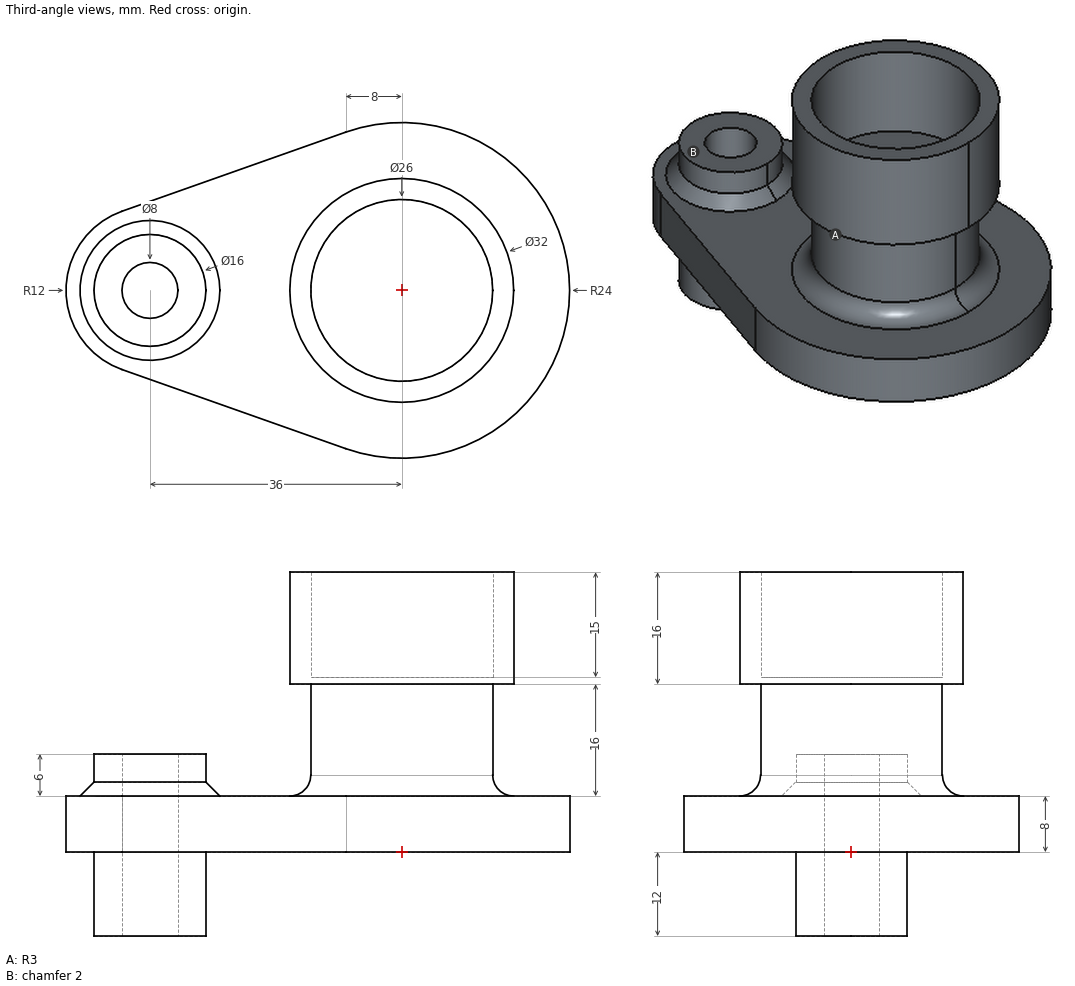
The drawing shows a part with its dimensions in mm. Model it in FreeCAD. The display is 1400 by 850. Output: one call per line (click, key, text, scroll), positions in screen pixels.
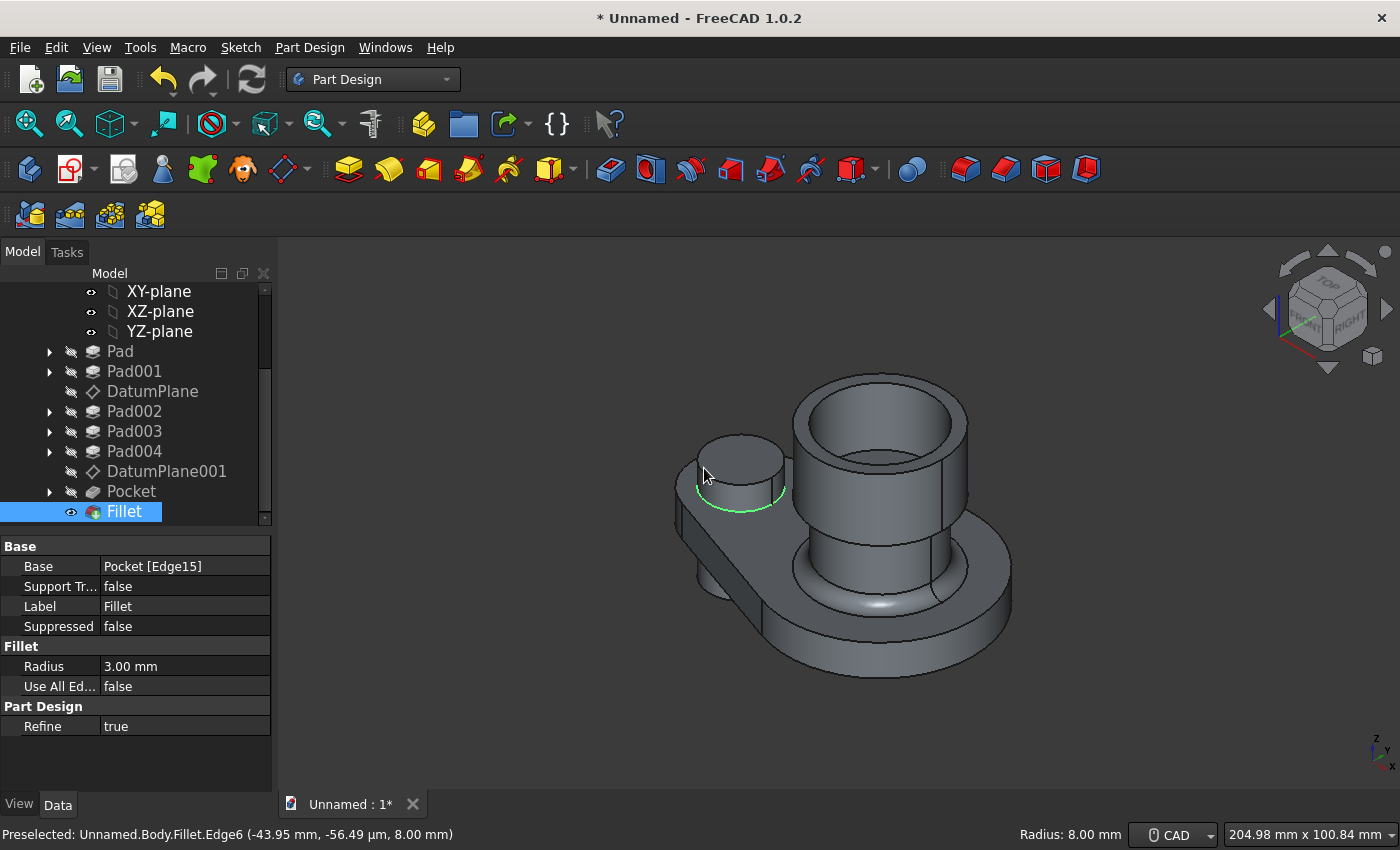
click(1006, 170)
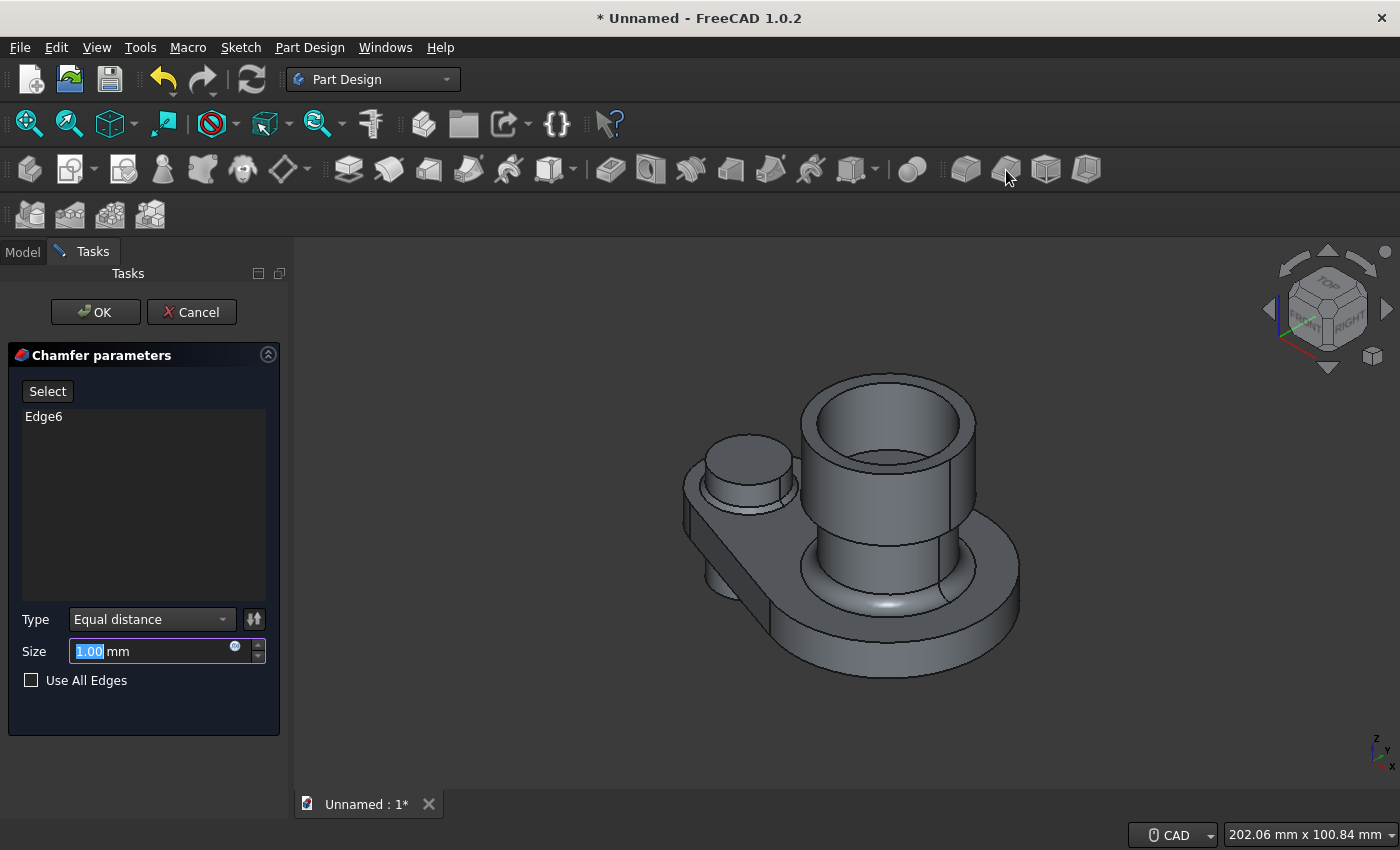
text(2)
key(Tab)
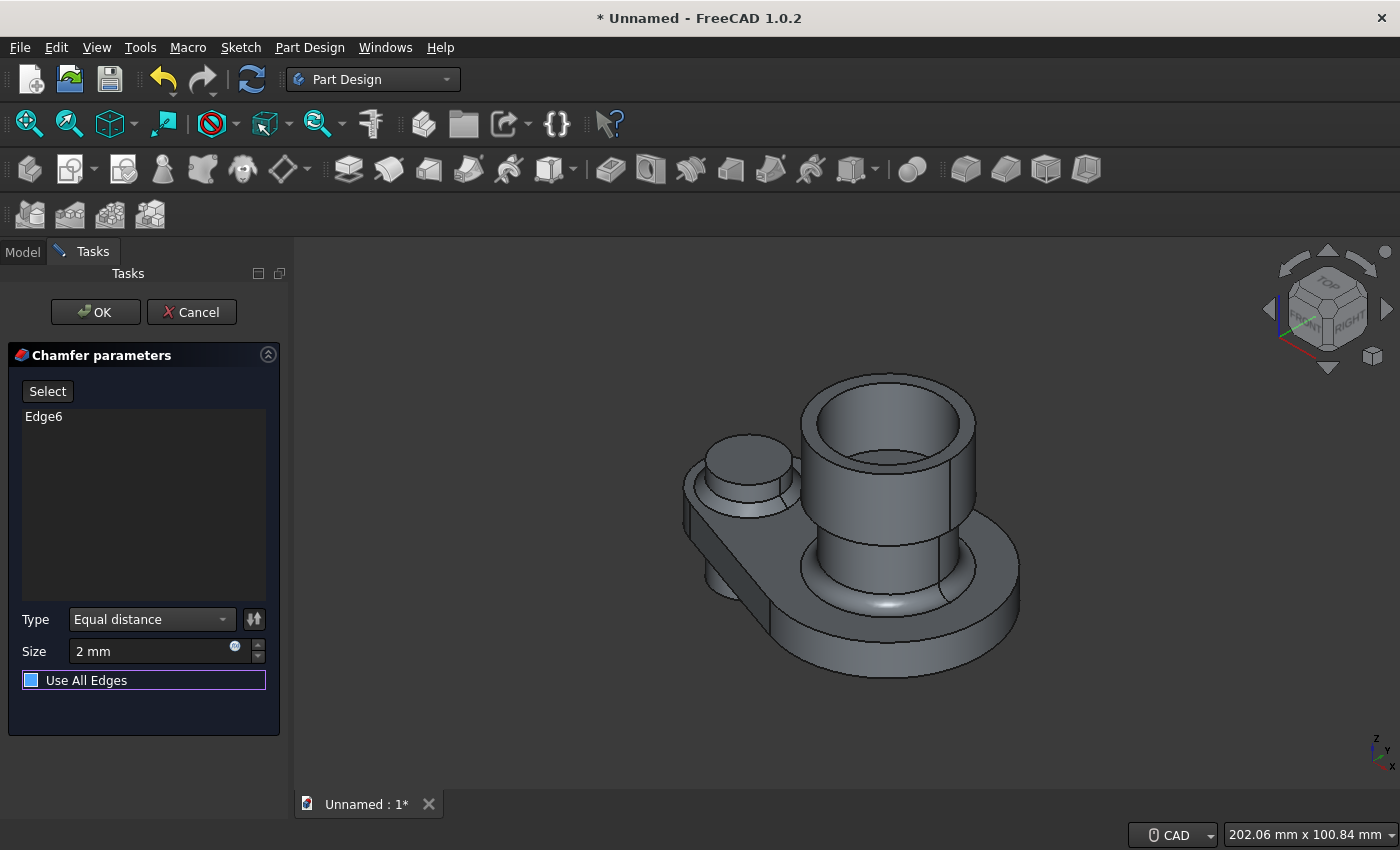
click(96, 312)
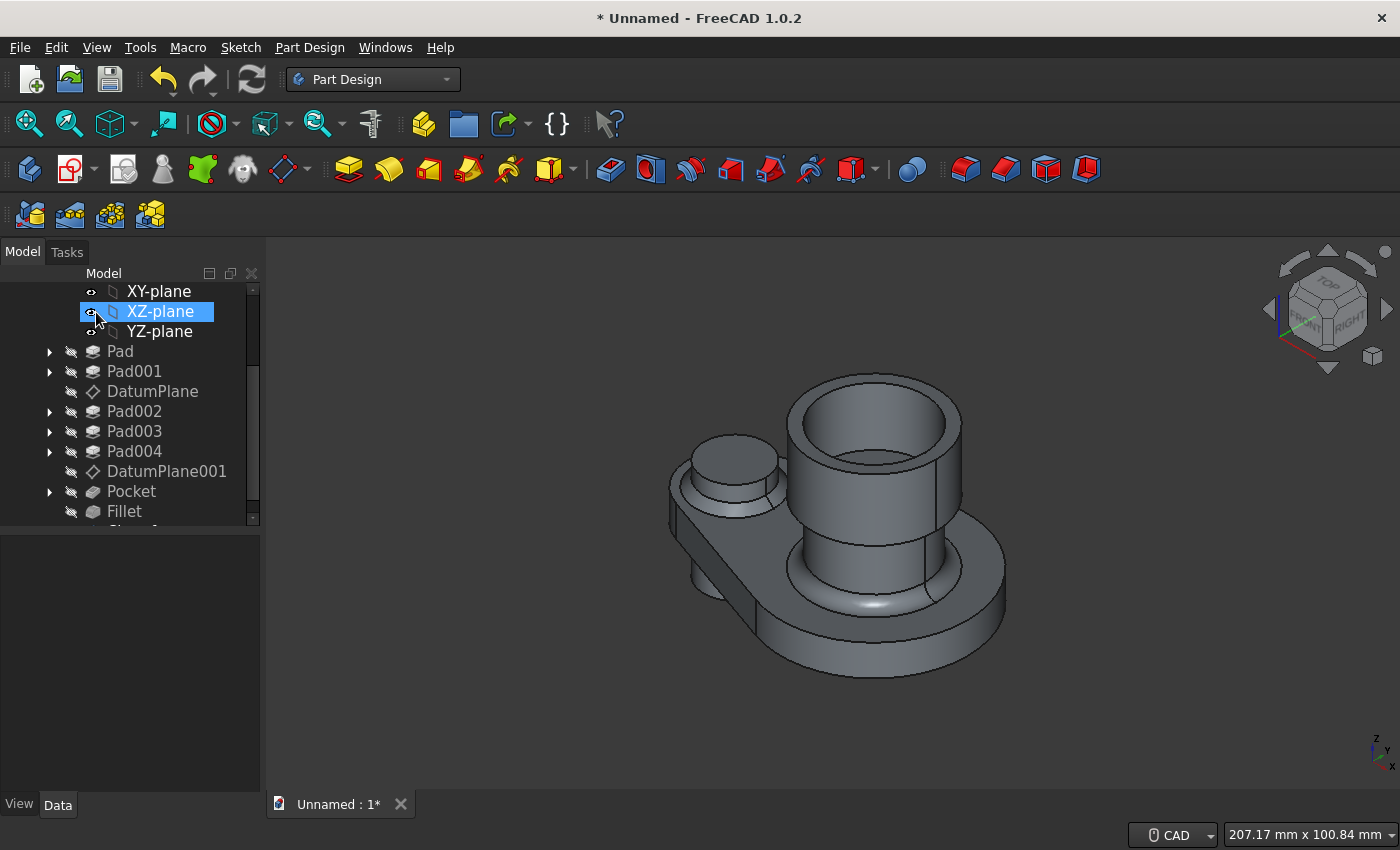
click(735, 459)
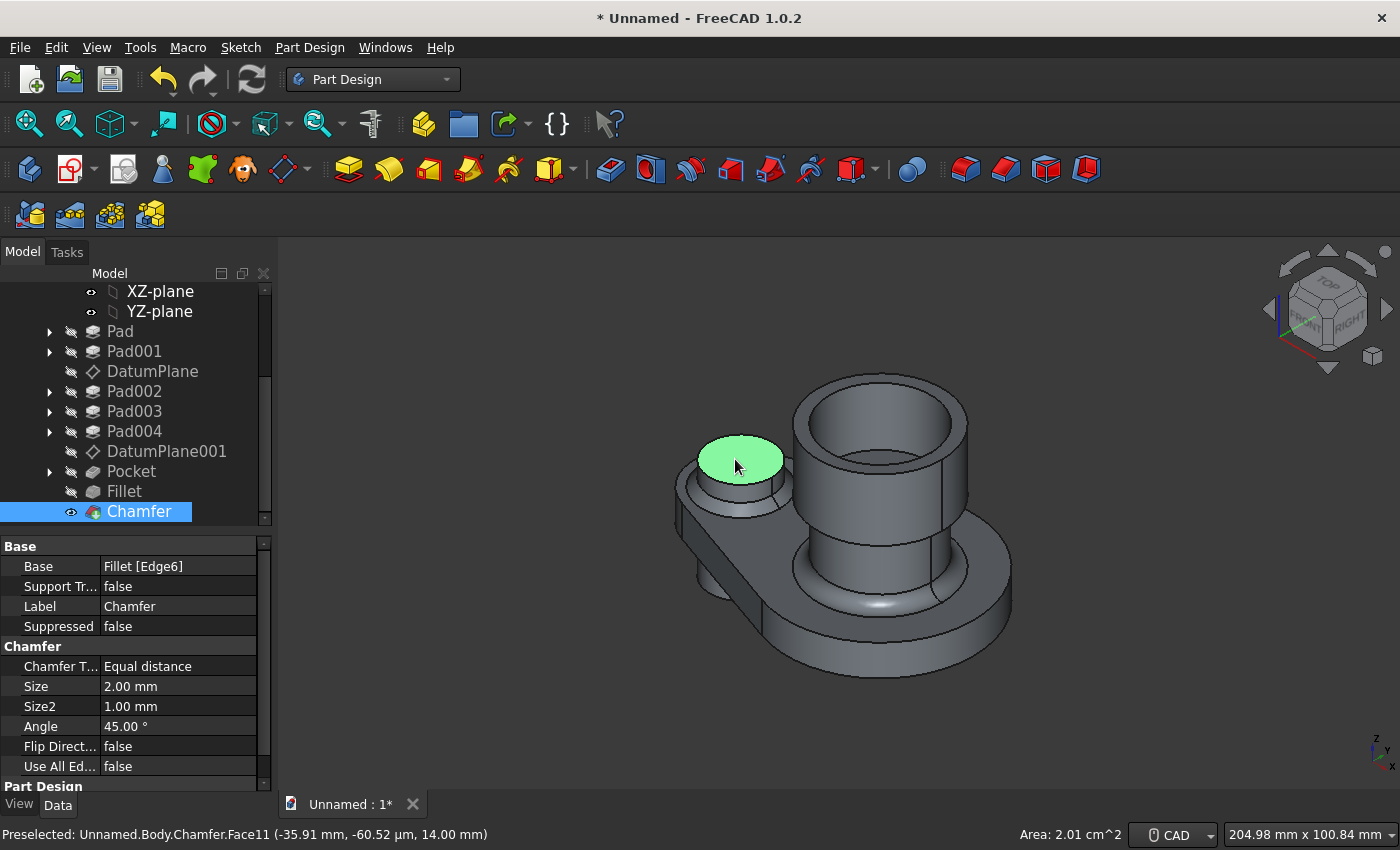
click(70, 170)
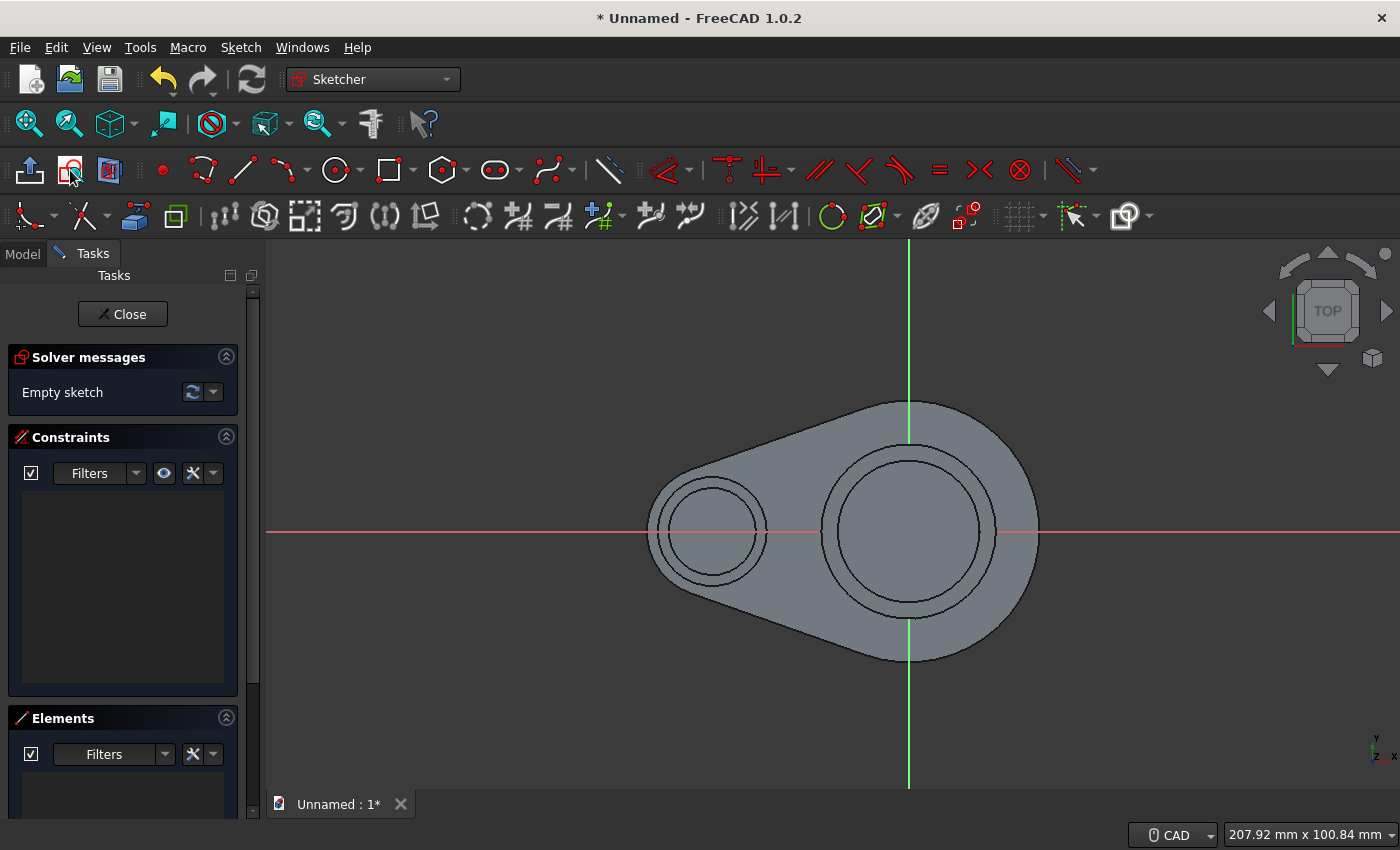
click(110, 170)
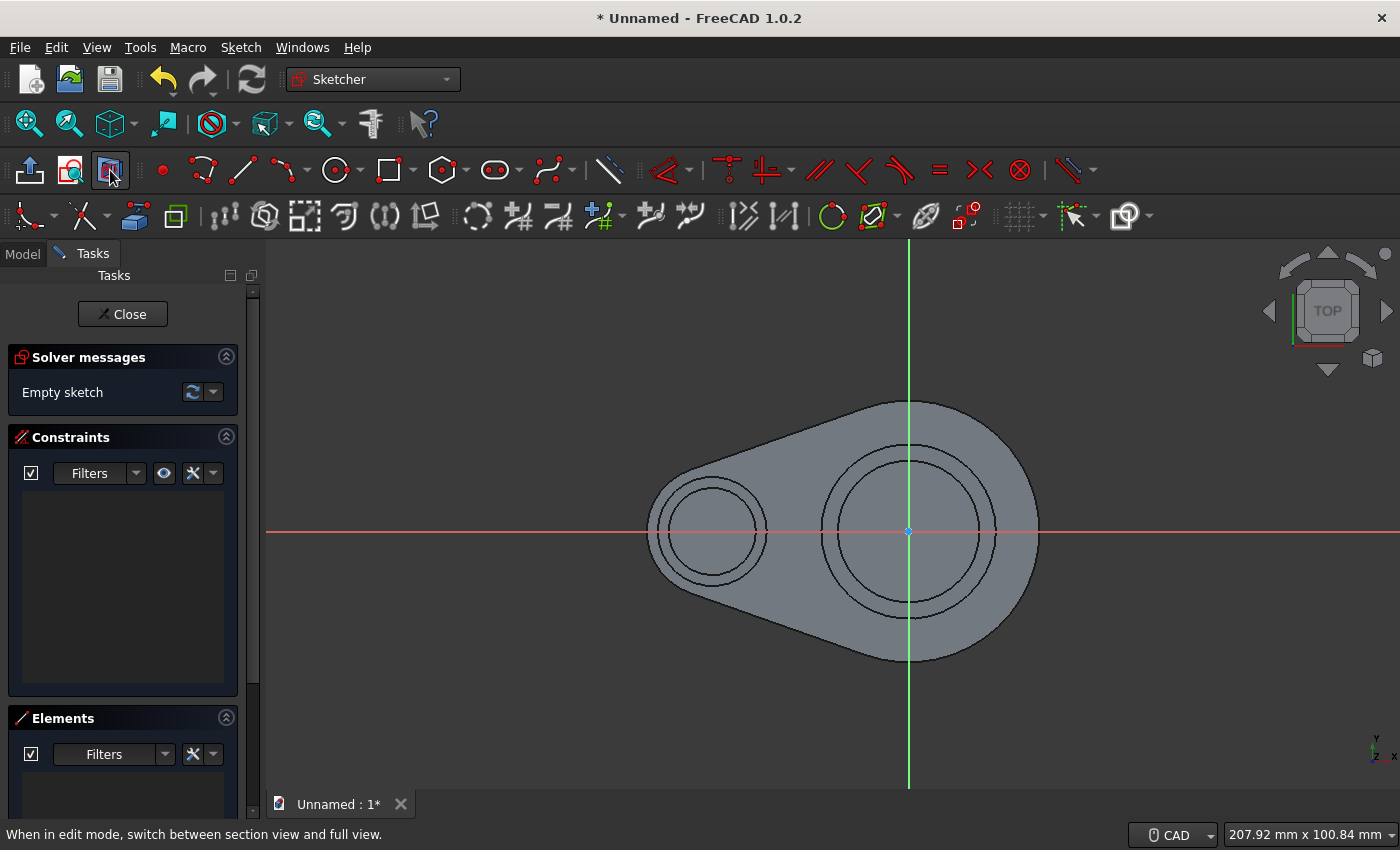
scroll(704, 534, up, 10)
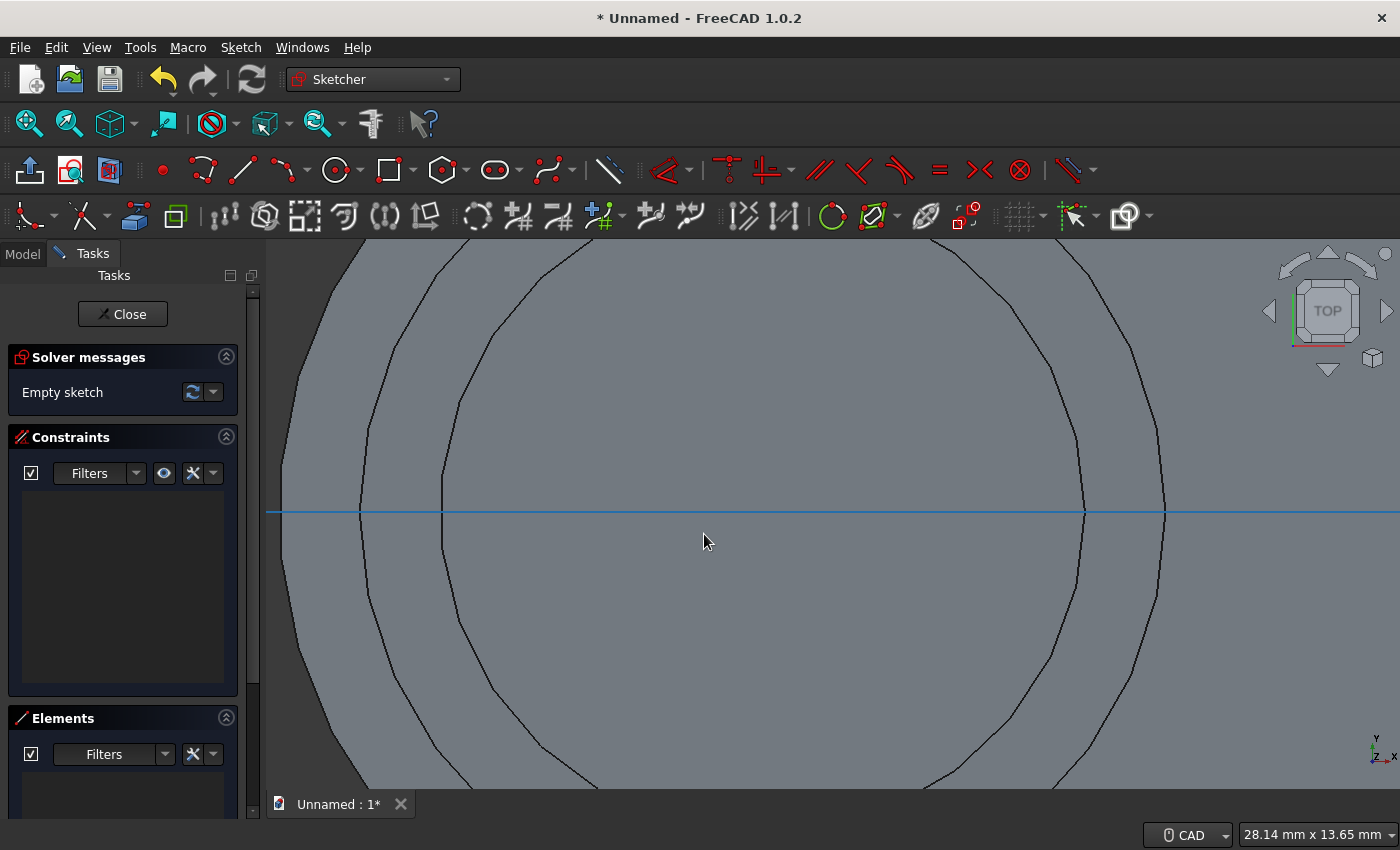
click(336, 170)